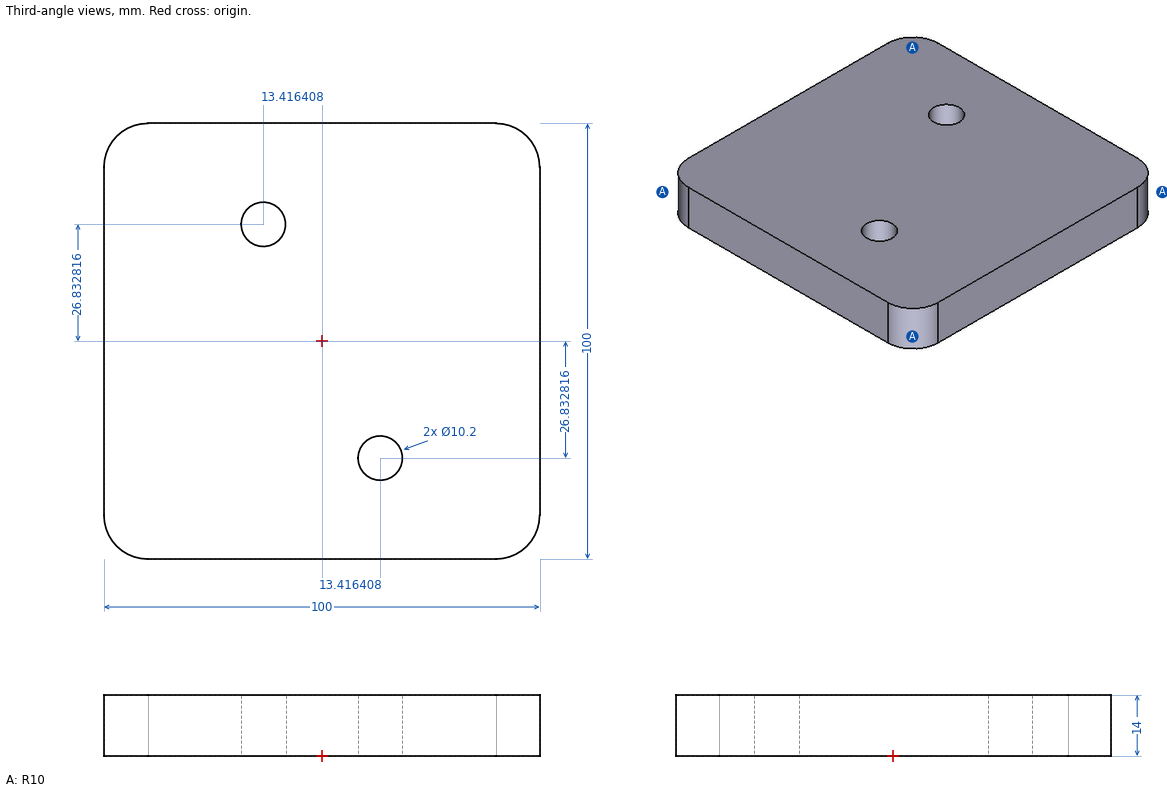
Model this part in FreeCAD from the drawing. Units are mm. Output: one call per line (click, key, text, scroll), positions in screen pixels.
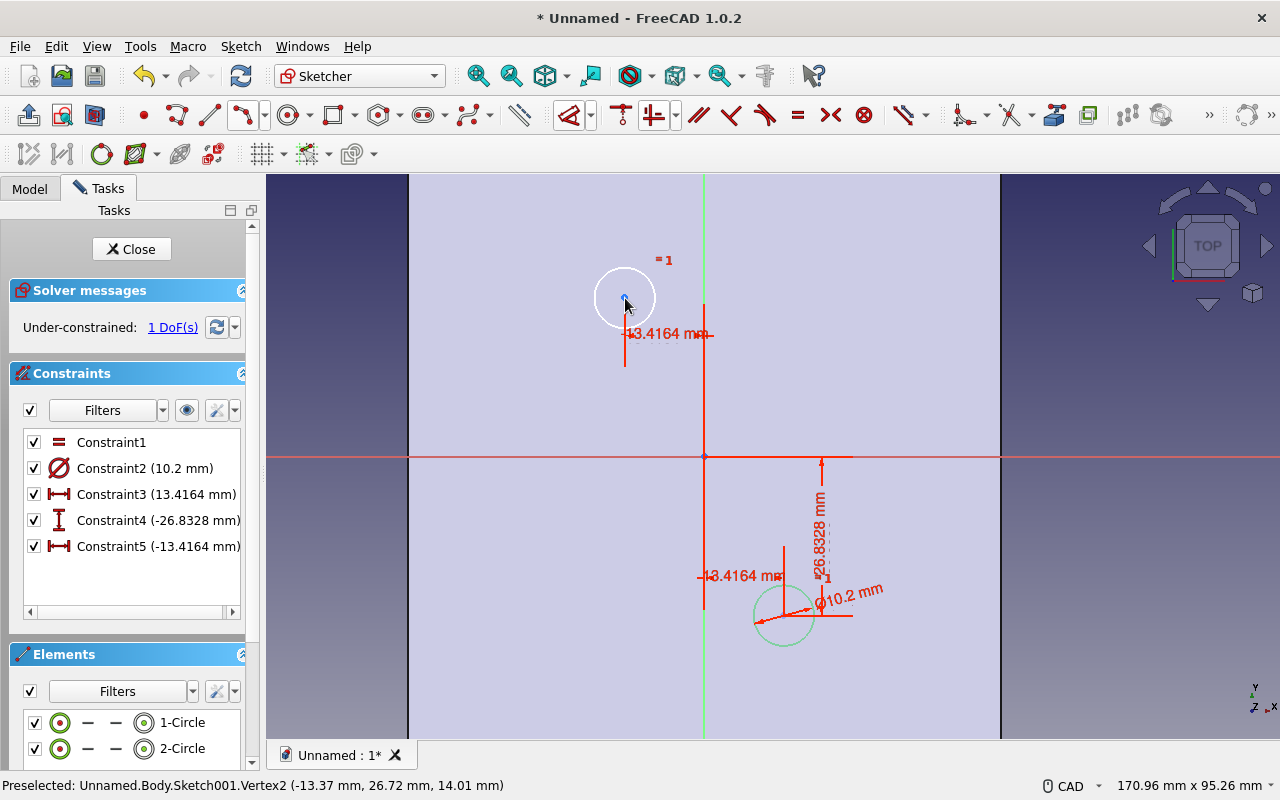
click(625, 298)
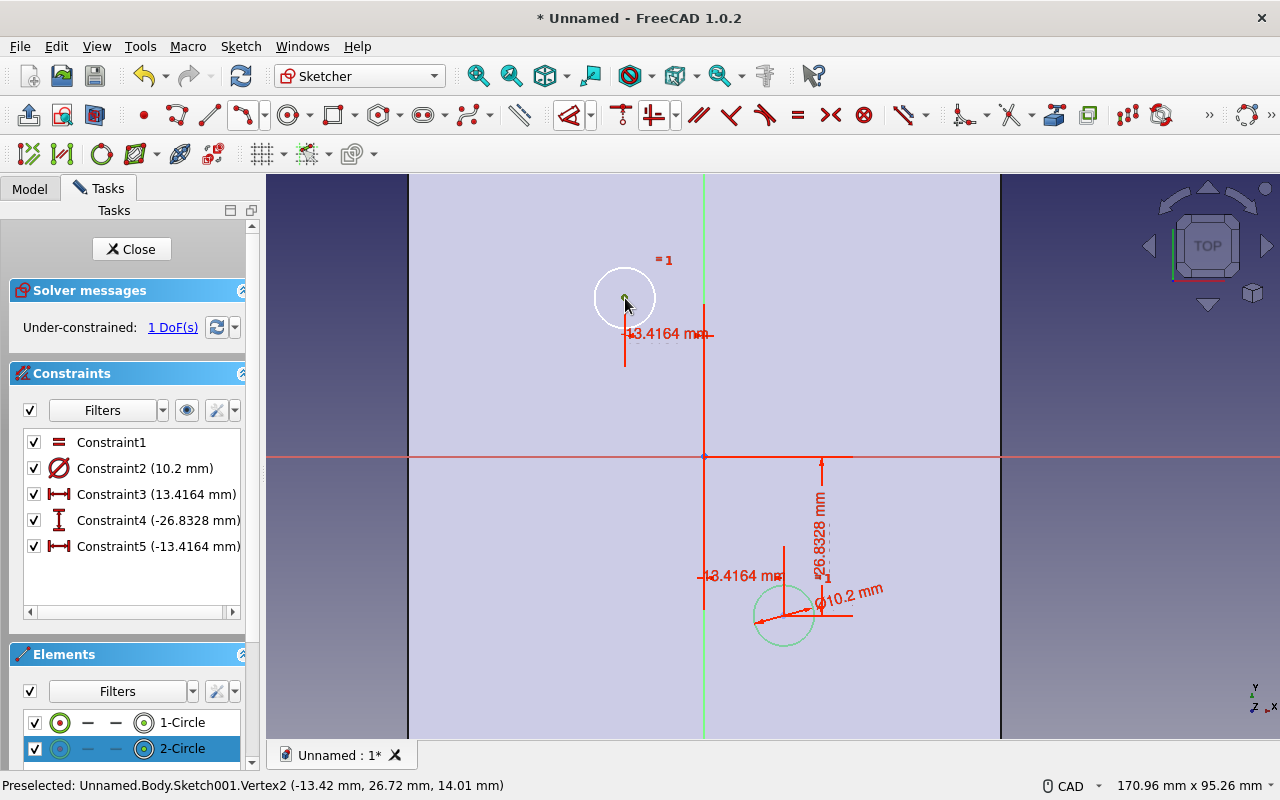
key(i)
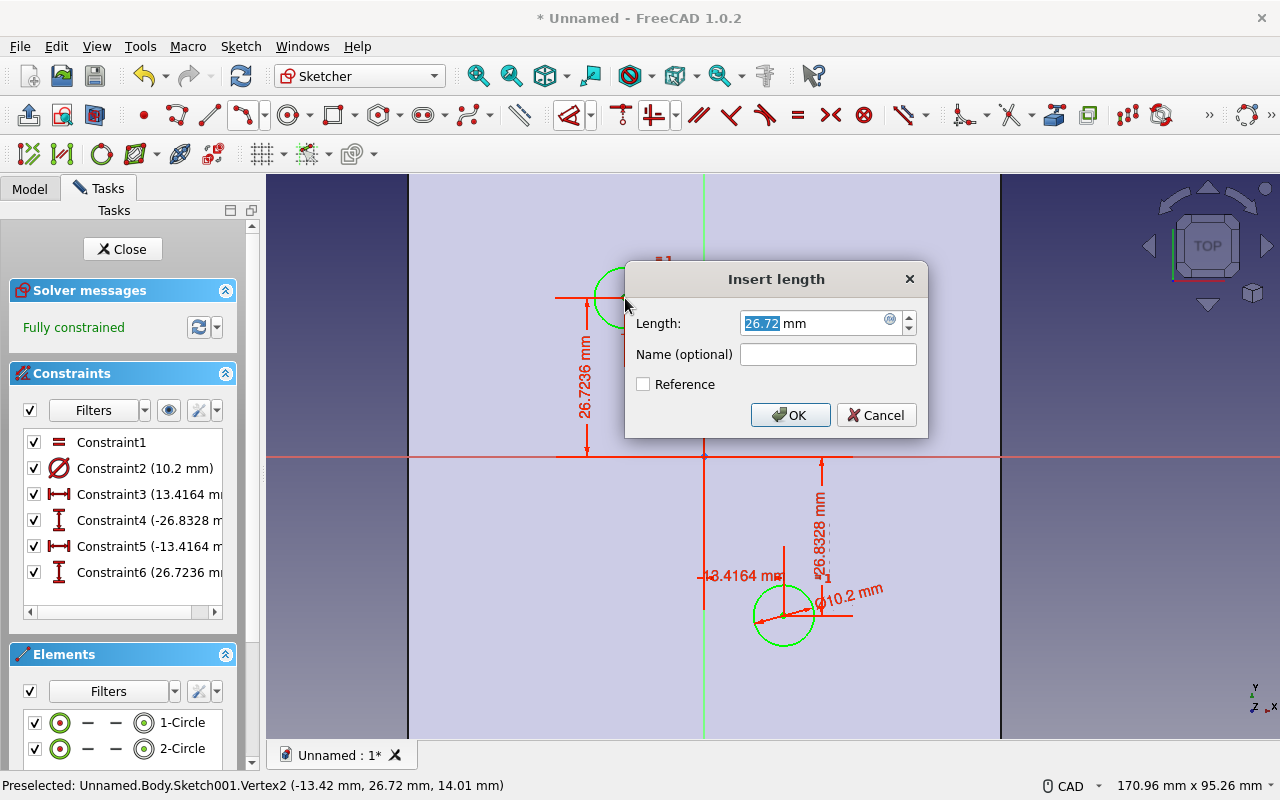
text(26.832816)
key(Return)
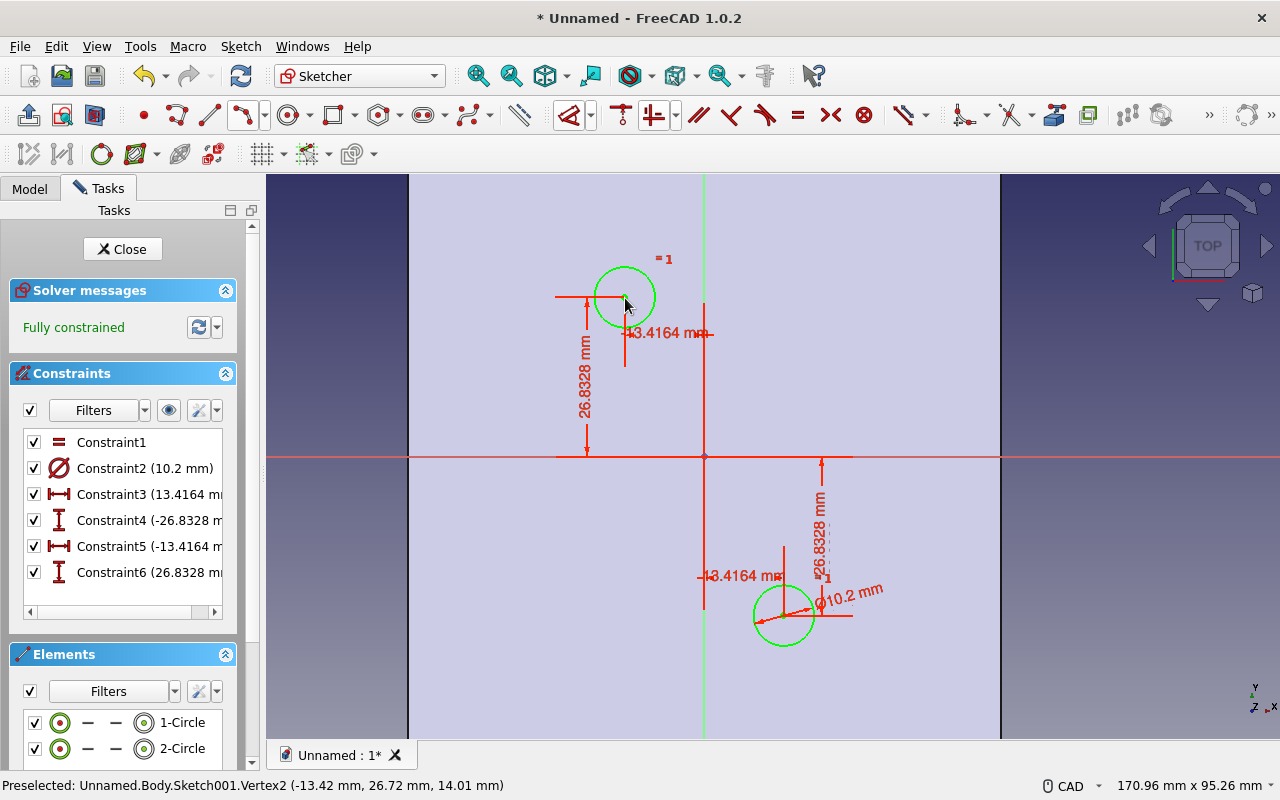
click(123, 249)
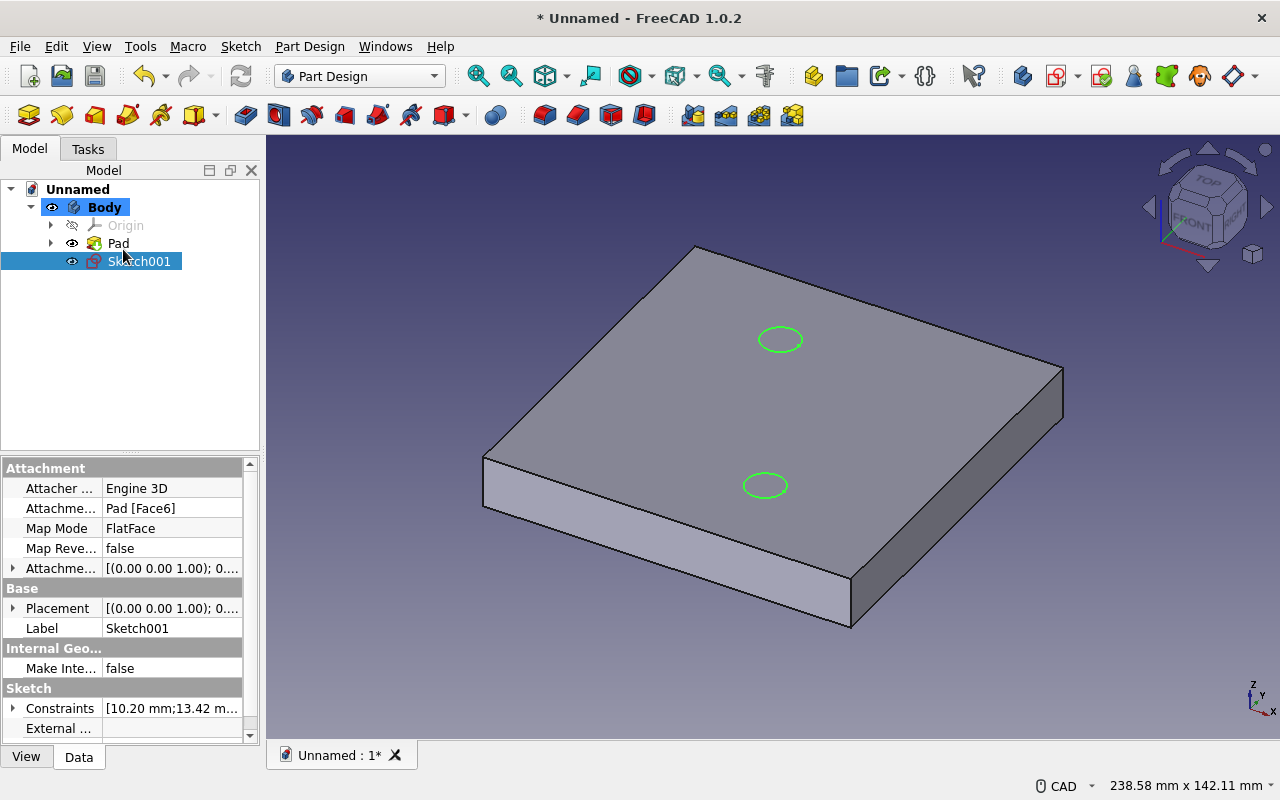
click(246, 116)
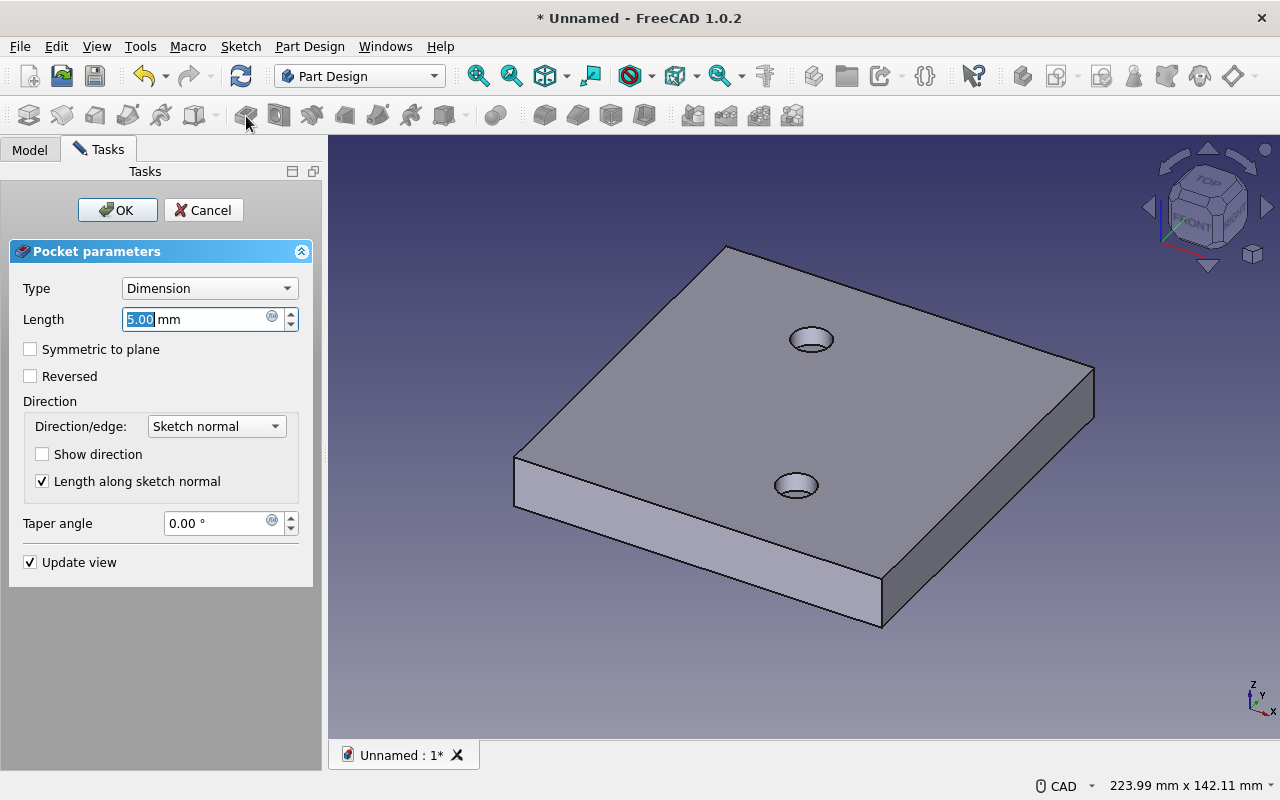
click(210, 288)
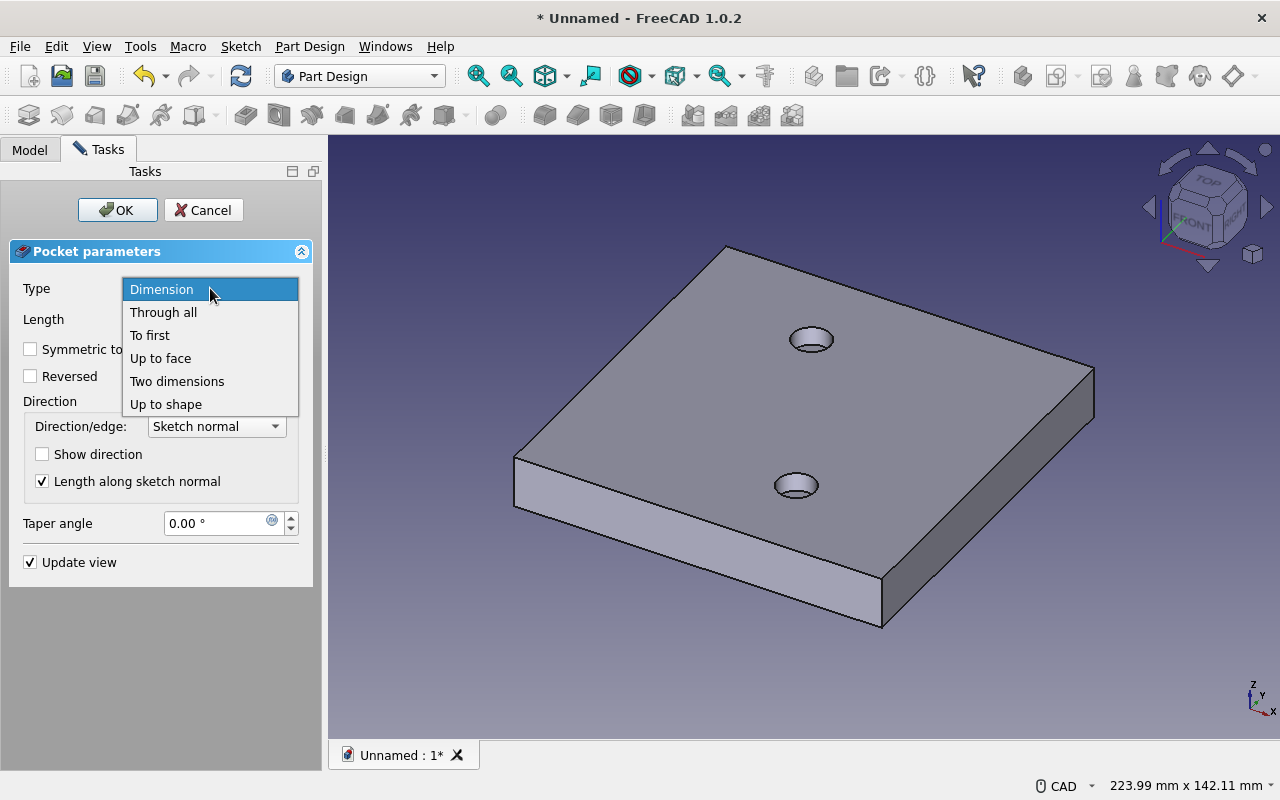
click(208, 312)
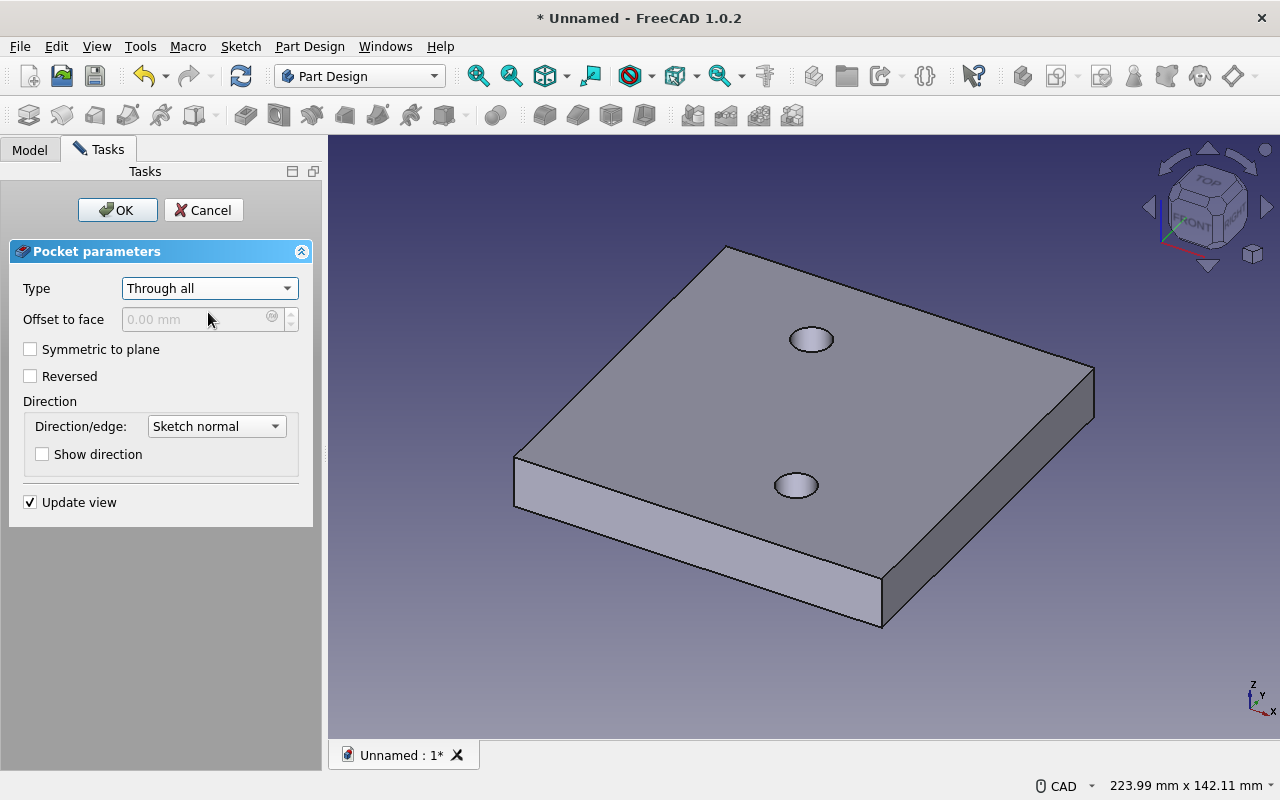
click(118, 210)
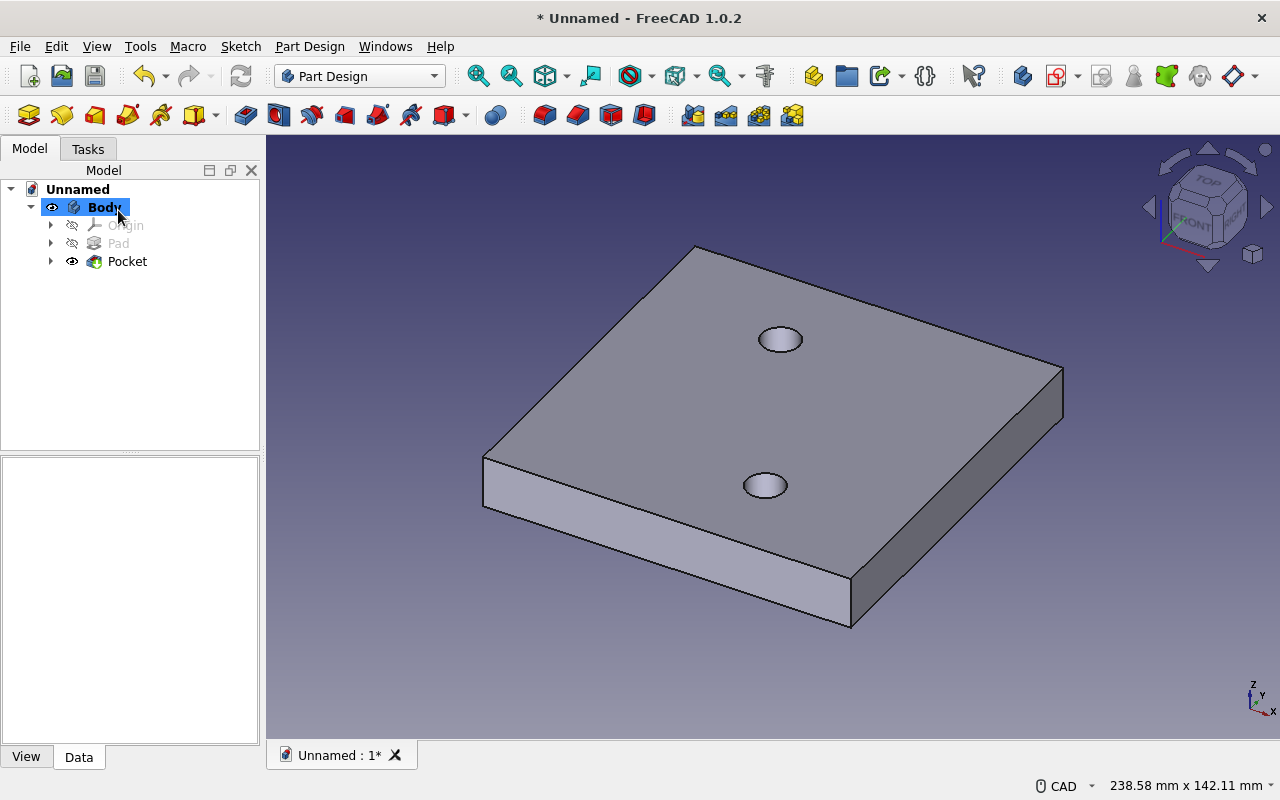
click(851, 603)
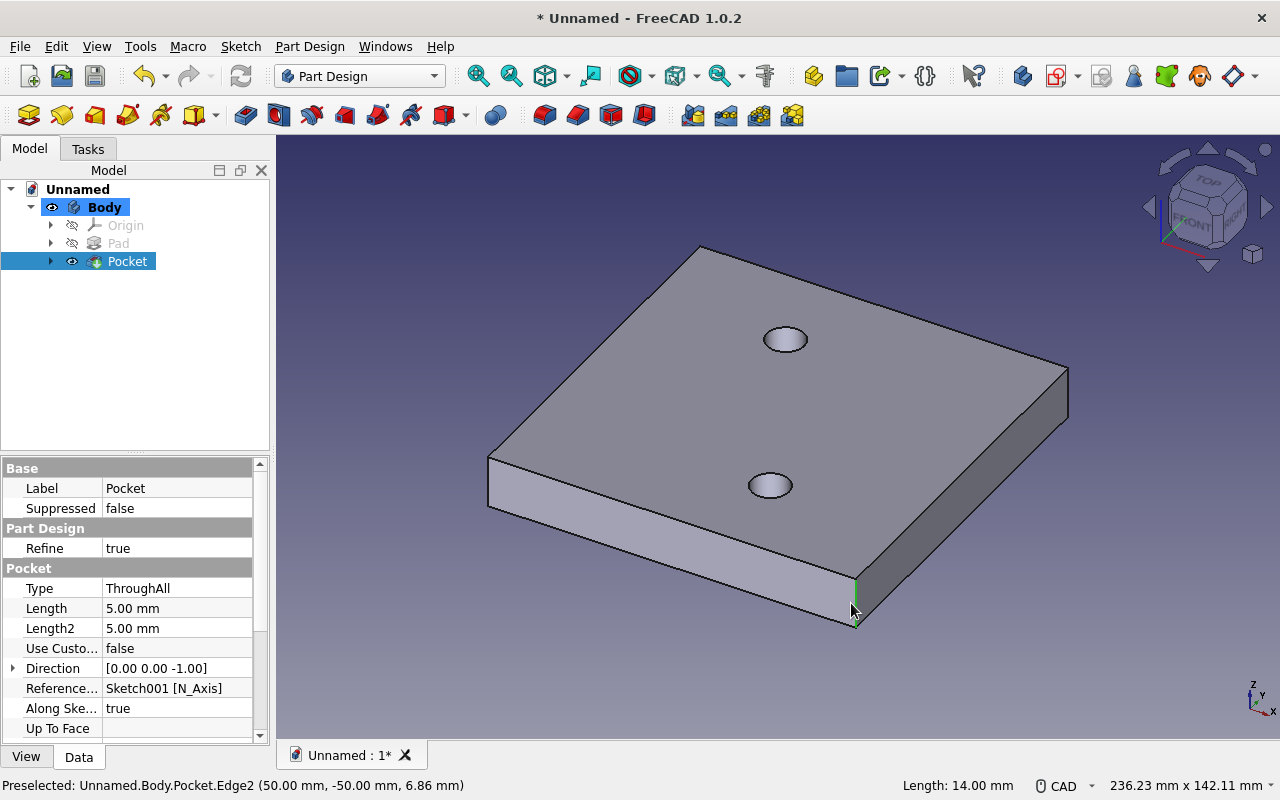
key(0)